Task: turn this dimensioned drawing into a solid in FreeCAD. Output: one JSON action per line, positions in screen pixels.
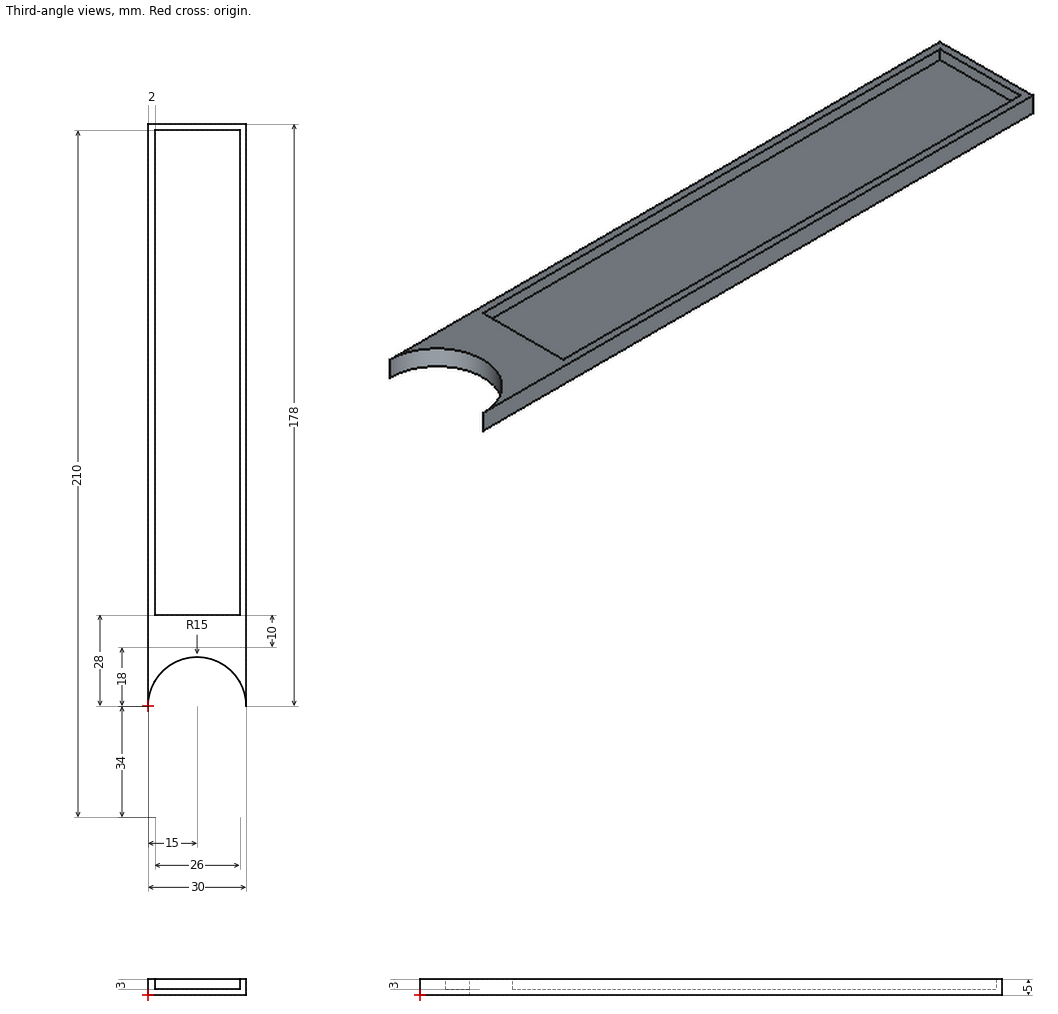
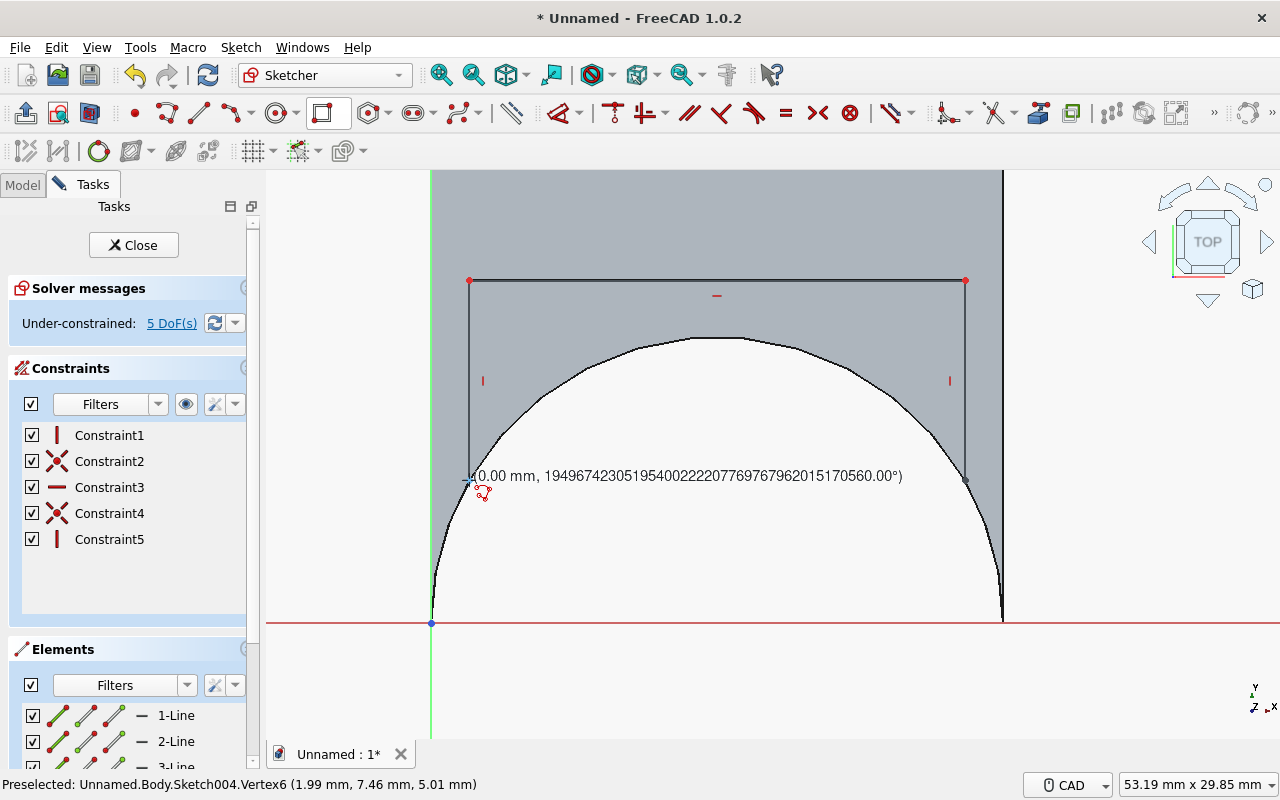
{"action": "key", "text": "g 3 a"}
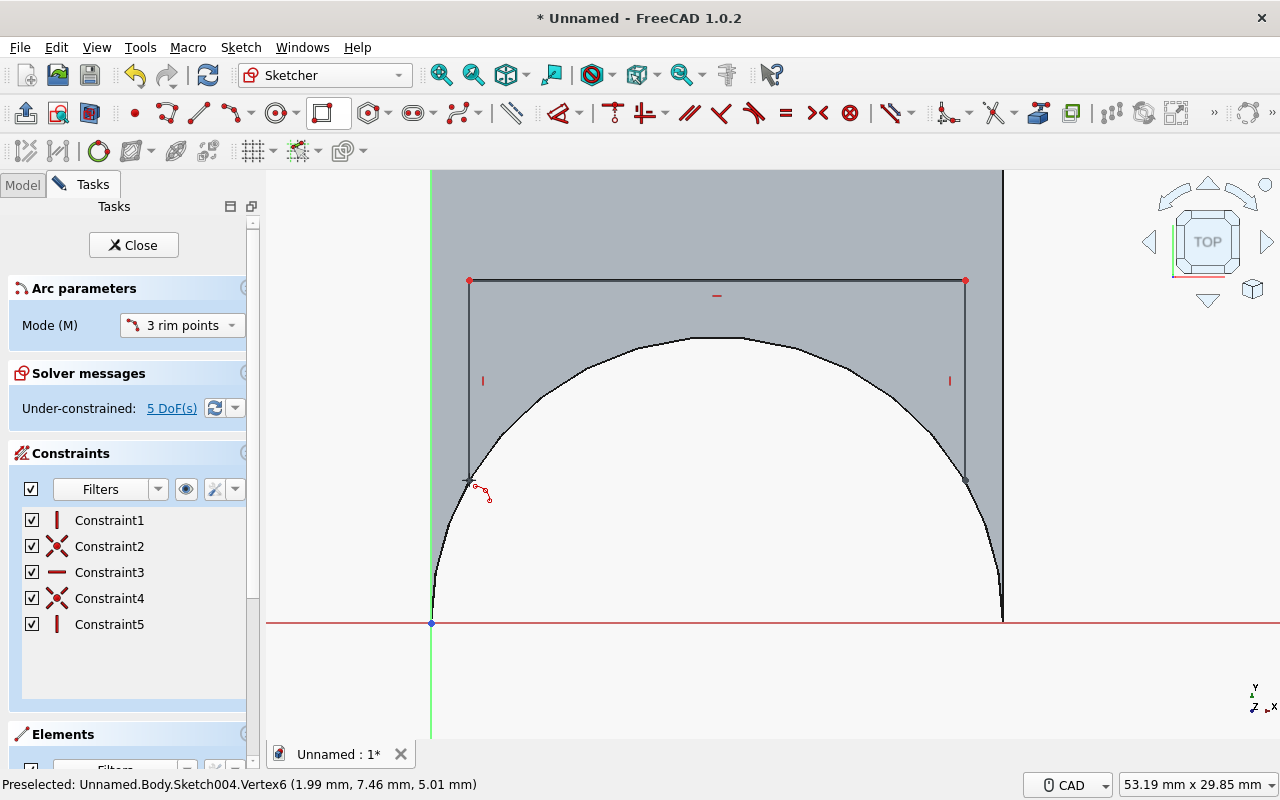
{"action": "left_click", "coordinate": [469, 481]}
{"action": "left_click", "coordinate": [965, 481]}
{"action": "left_click", "coordinate": [717, 337]}
{"action": "key", "text": "Escape"}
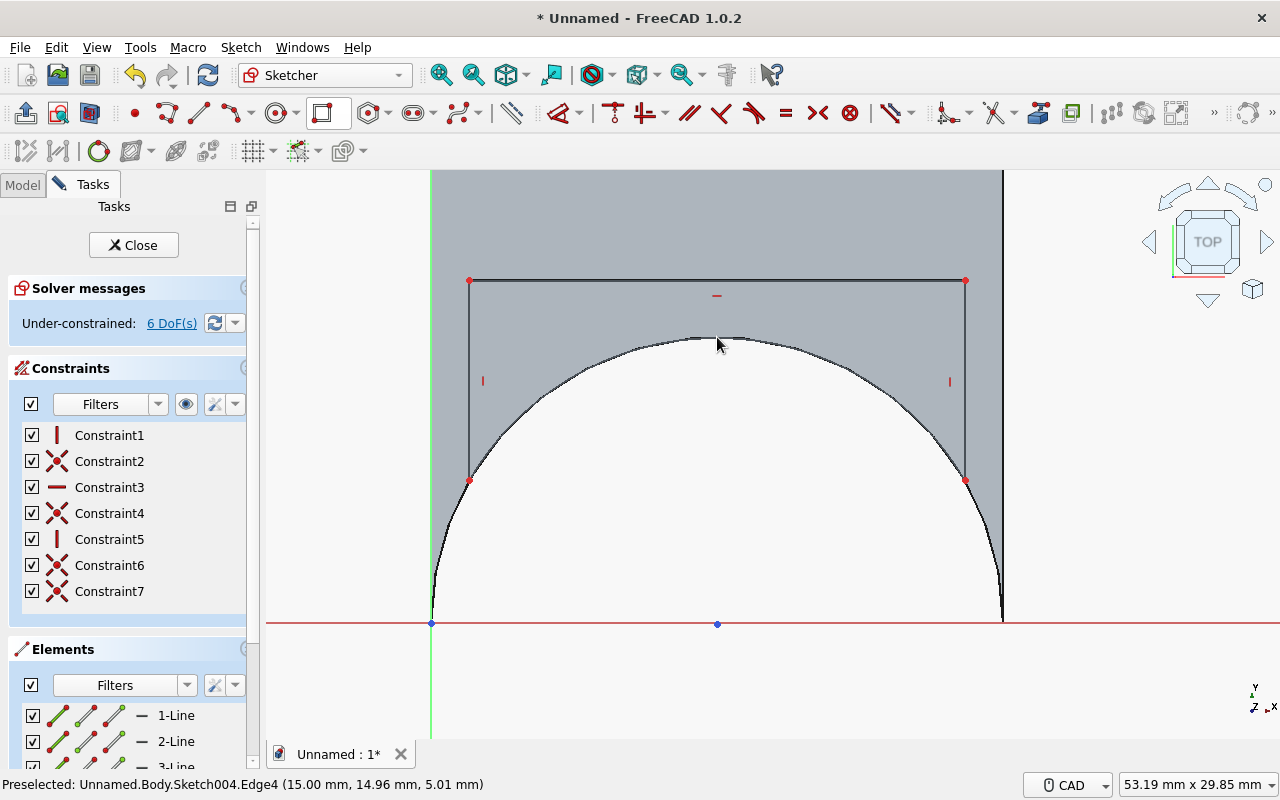
{"action": "left_click", "coordinate": [717, 625]}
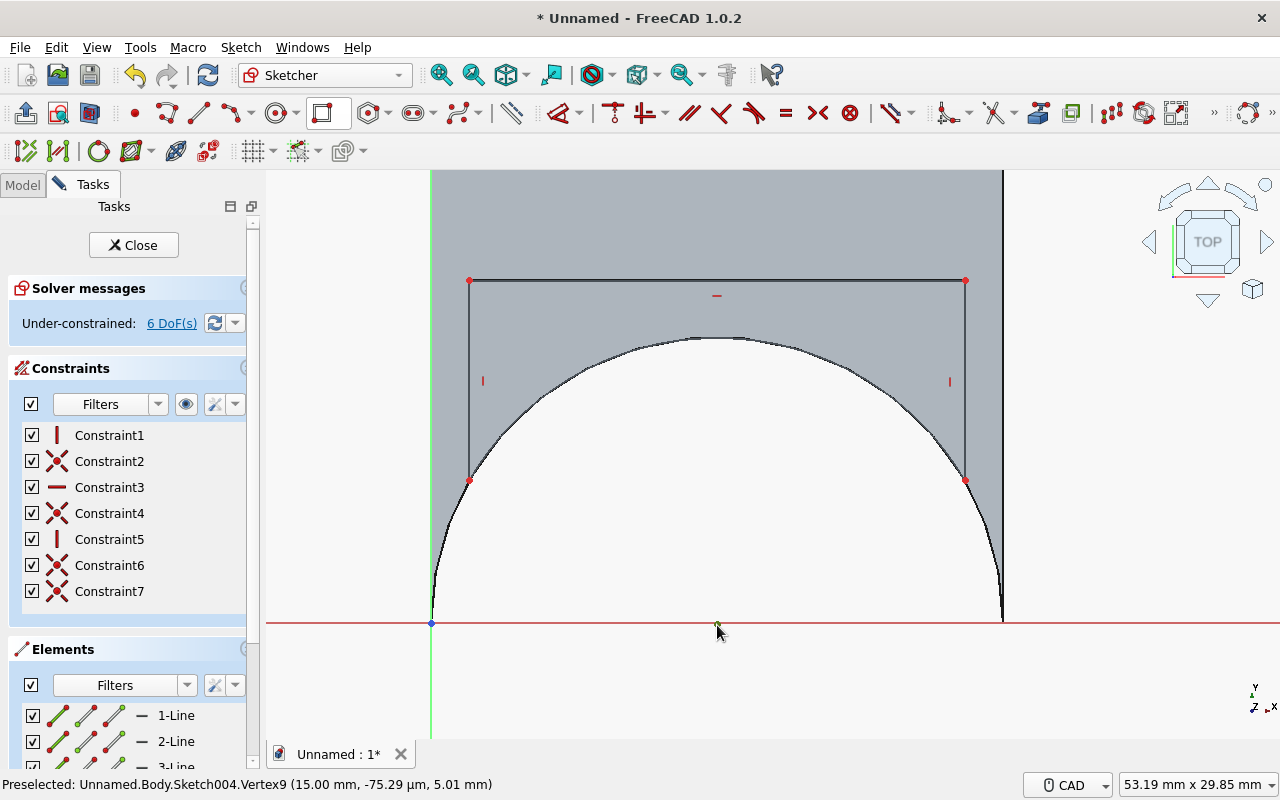
{"action": "left_click", "coordinate": [353, 623]}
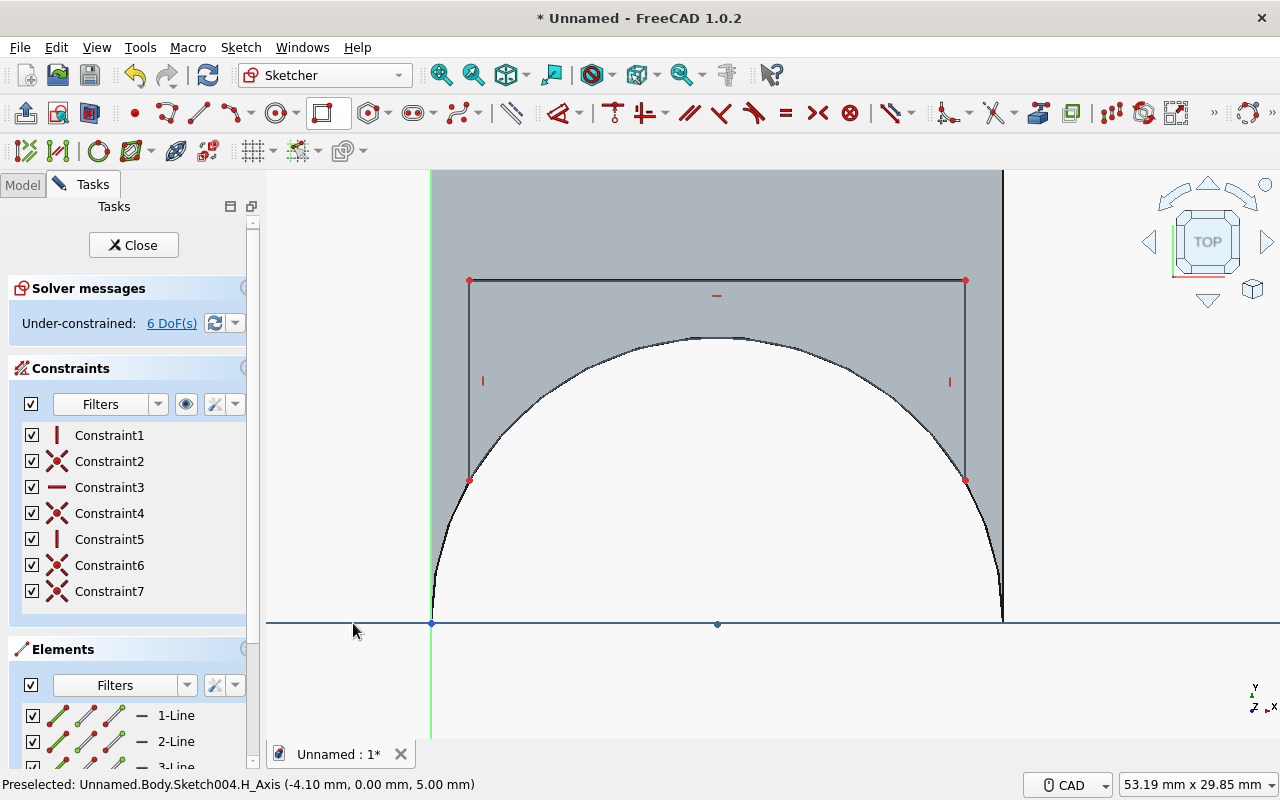
{"action": "key", "text": "c"}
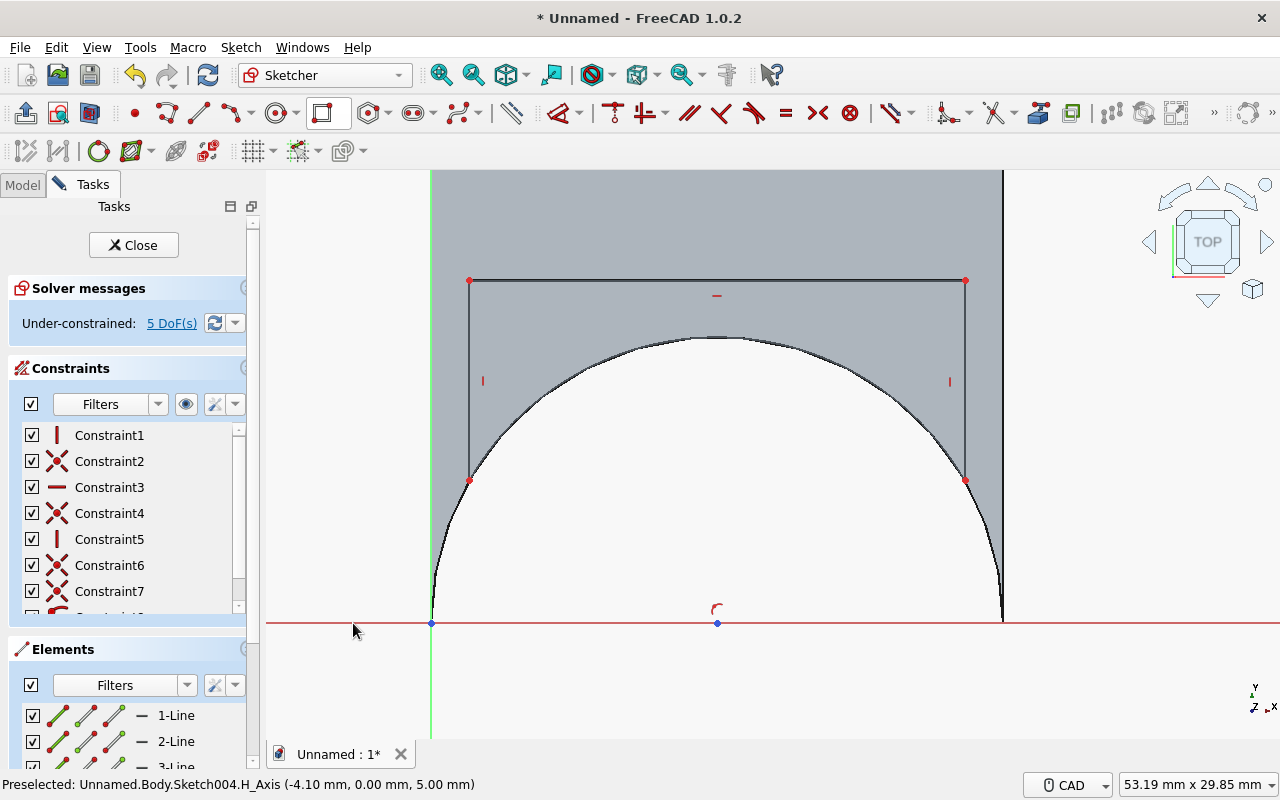
{"action": "left_click", "coordinate": [834, 362]}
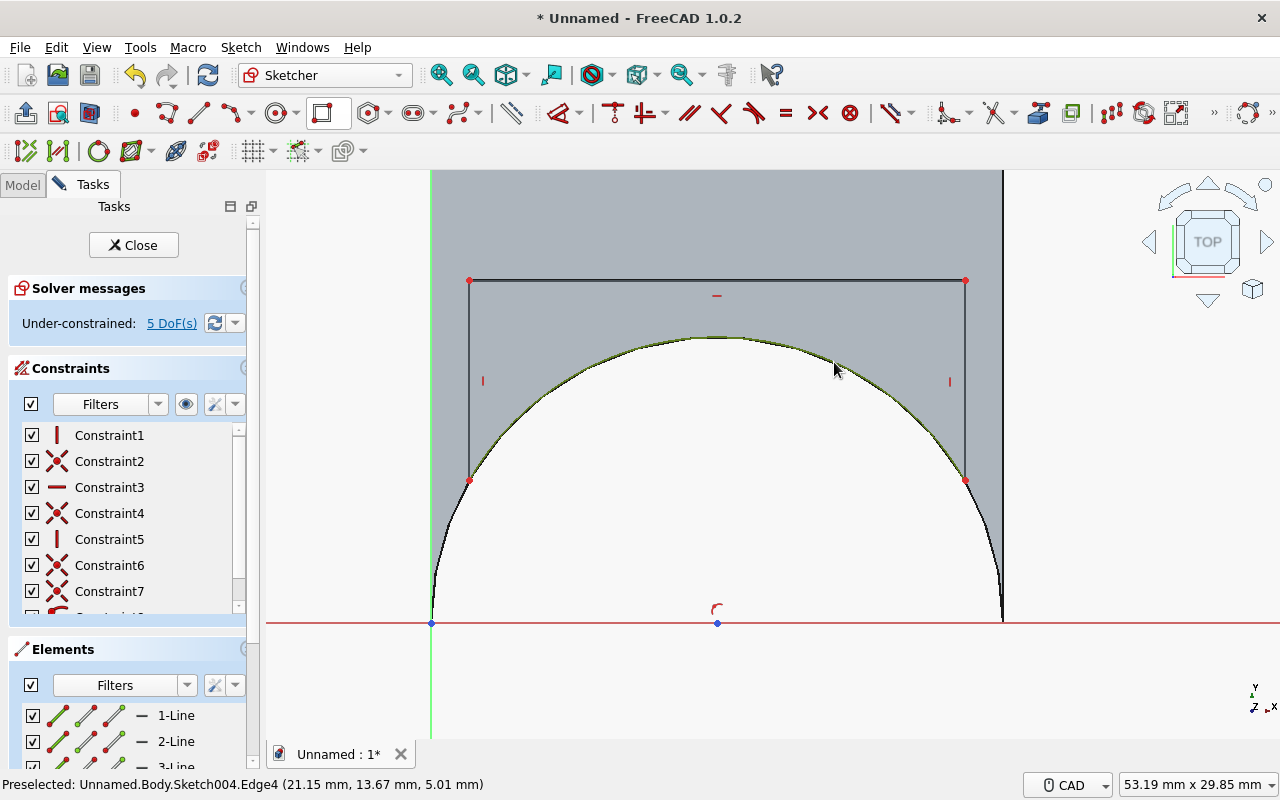
{"action": "left_click", "coordinate": [582, 114]}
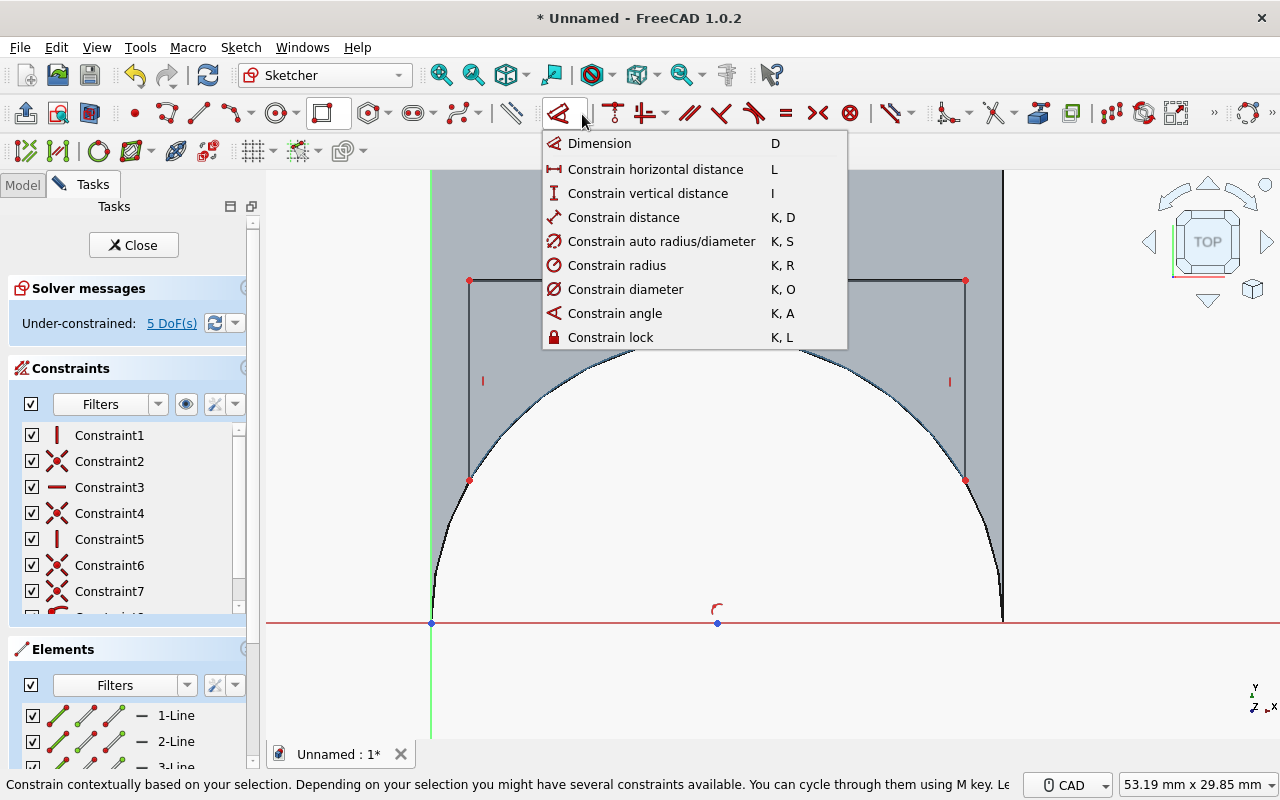
{"action": "left_click", "coordinate": [695, 265]}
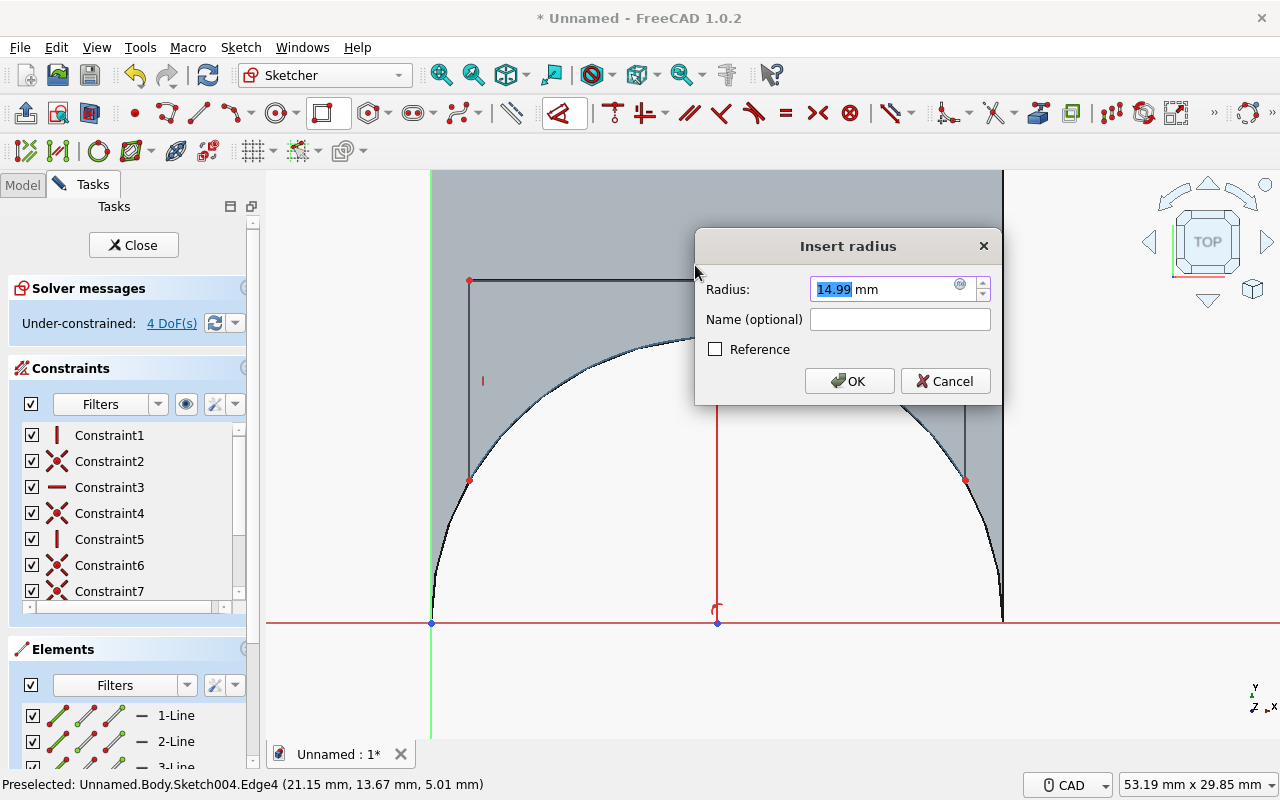
{"action": "type", "text": "15"}
{"action": "key", "text": "Return"}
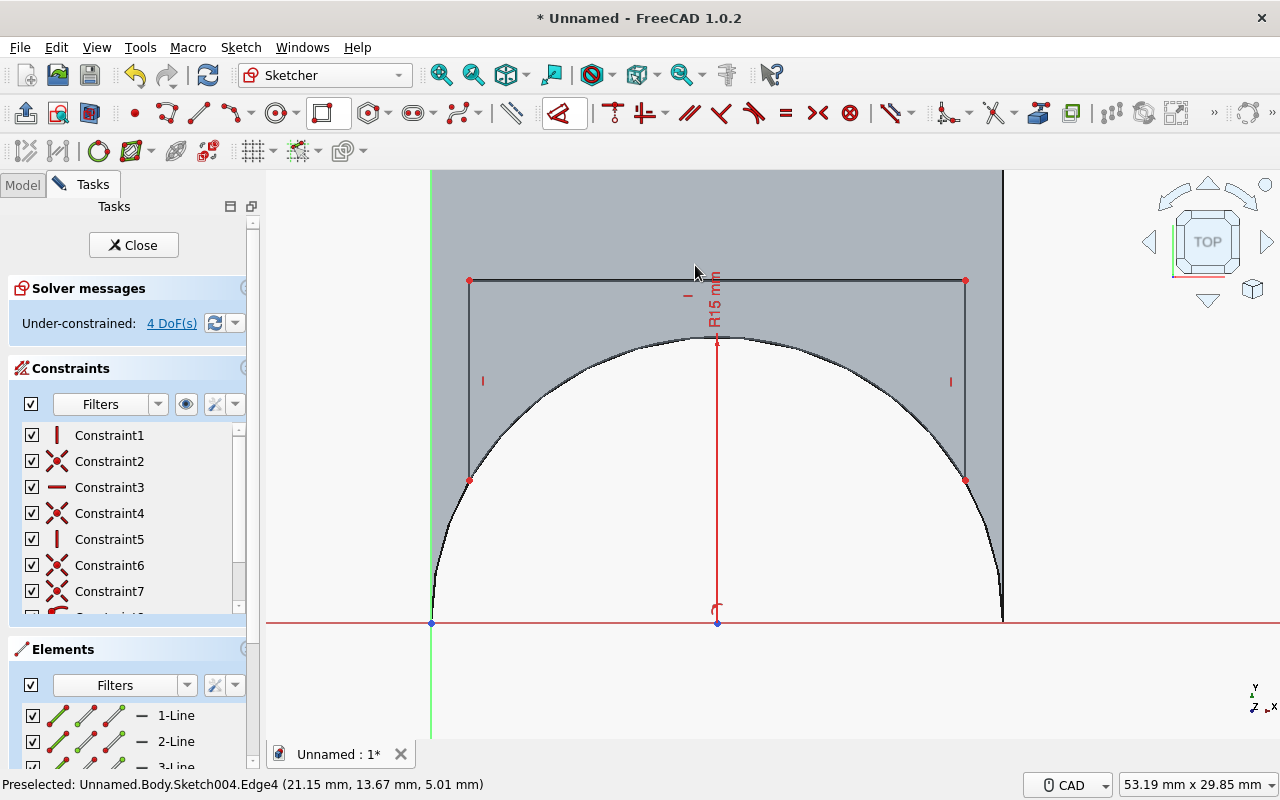
{"action": "left_click", "coordinate": [816, 281]}